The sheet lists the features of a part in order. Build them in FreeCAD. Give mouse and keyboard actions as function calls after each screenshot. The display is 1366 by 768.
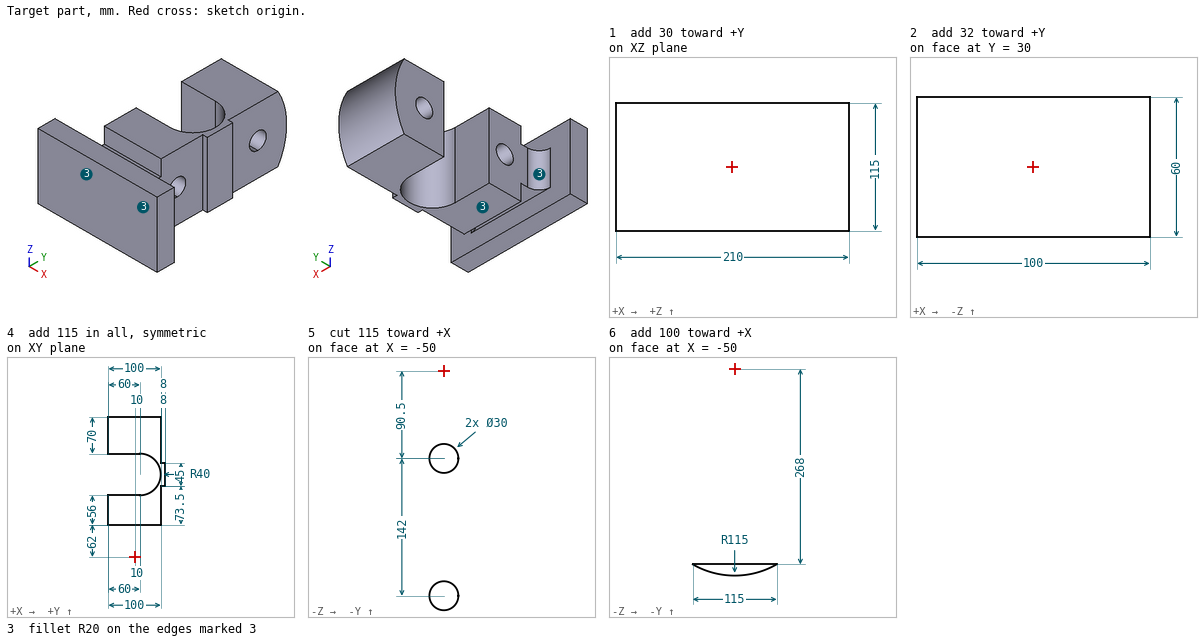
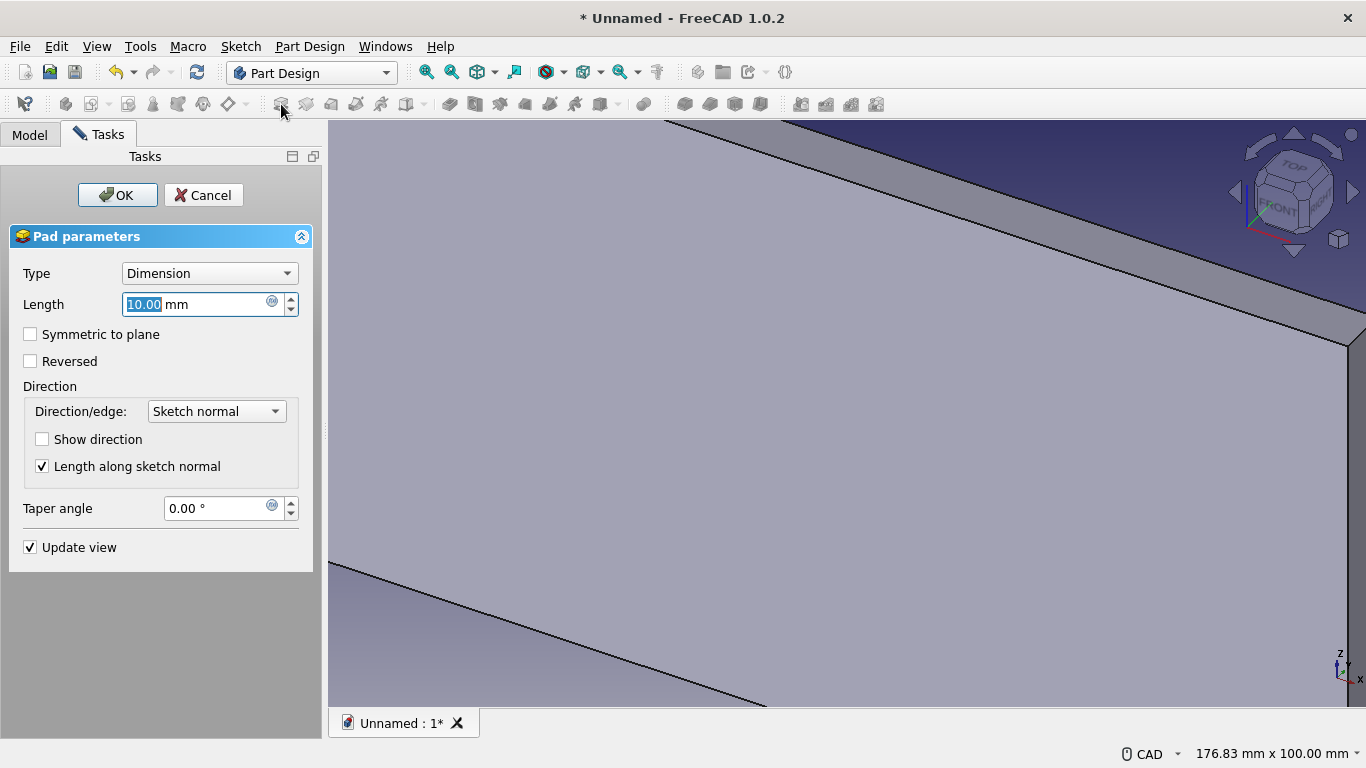
text(30)
key(Tab)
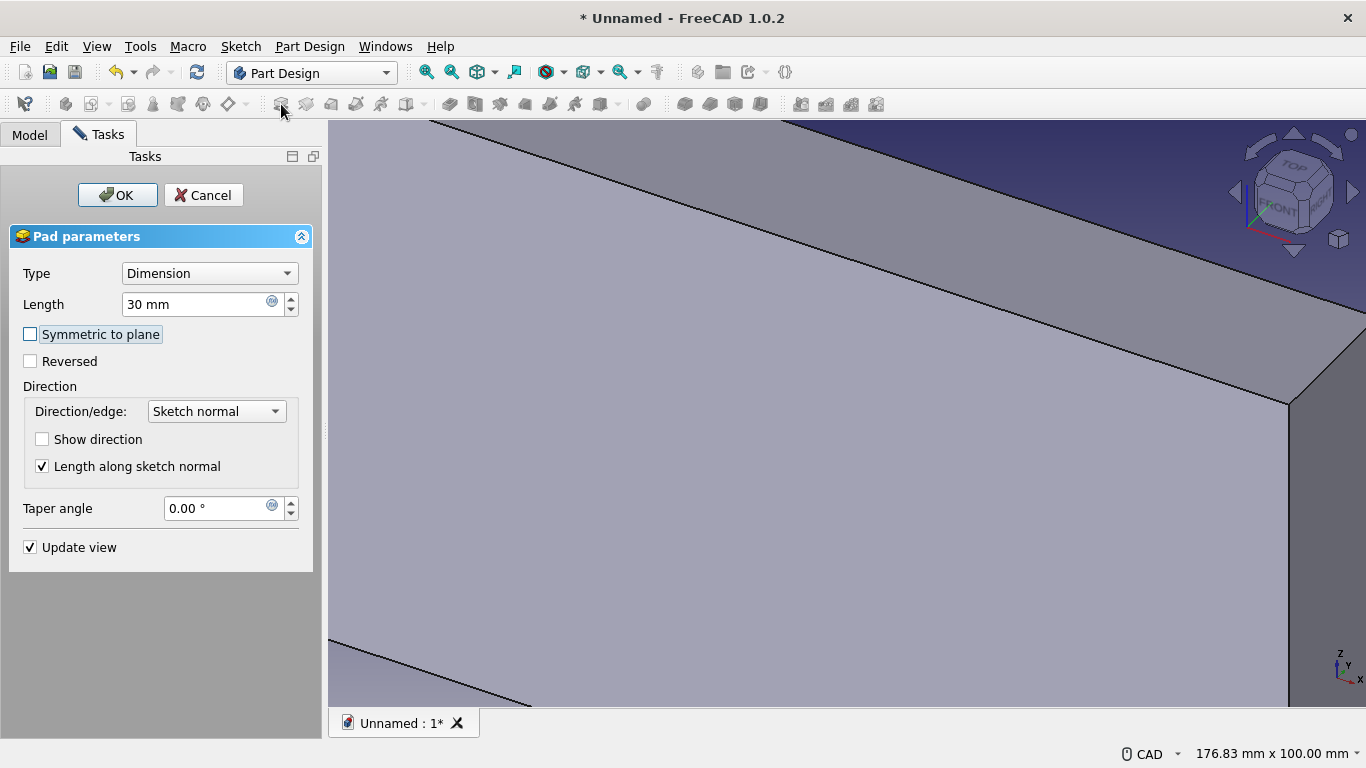
click(31, 361)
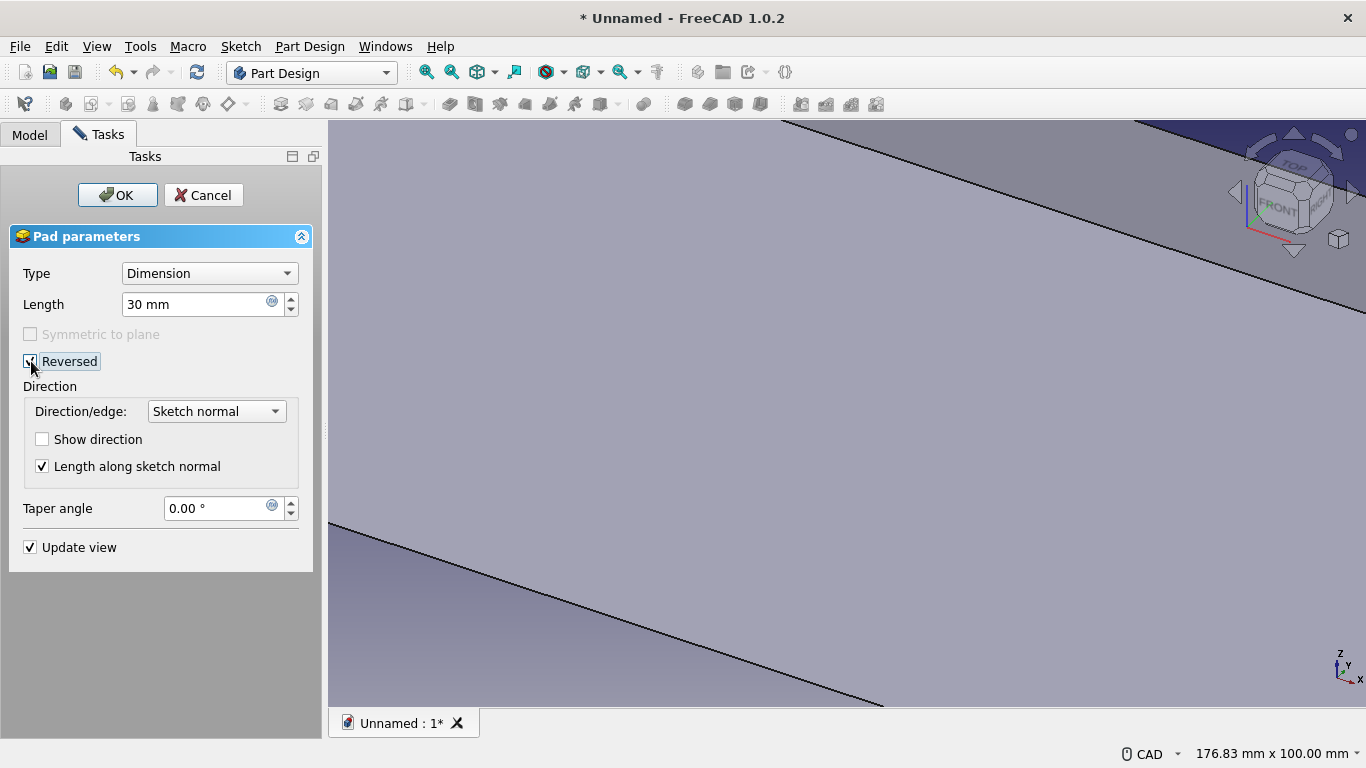
click(118, 195)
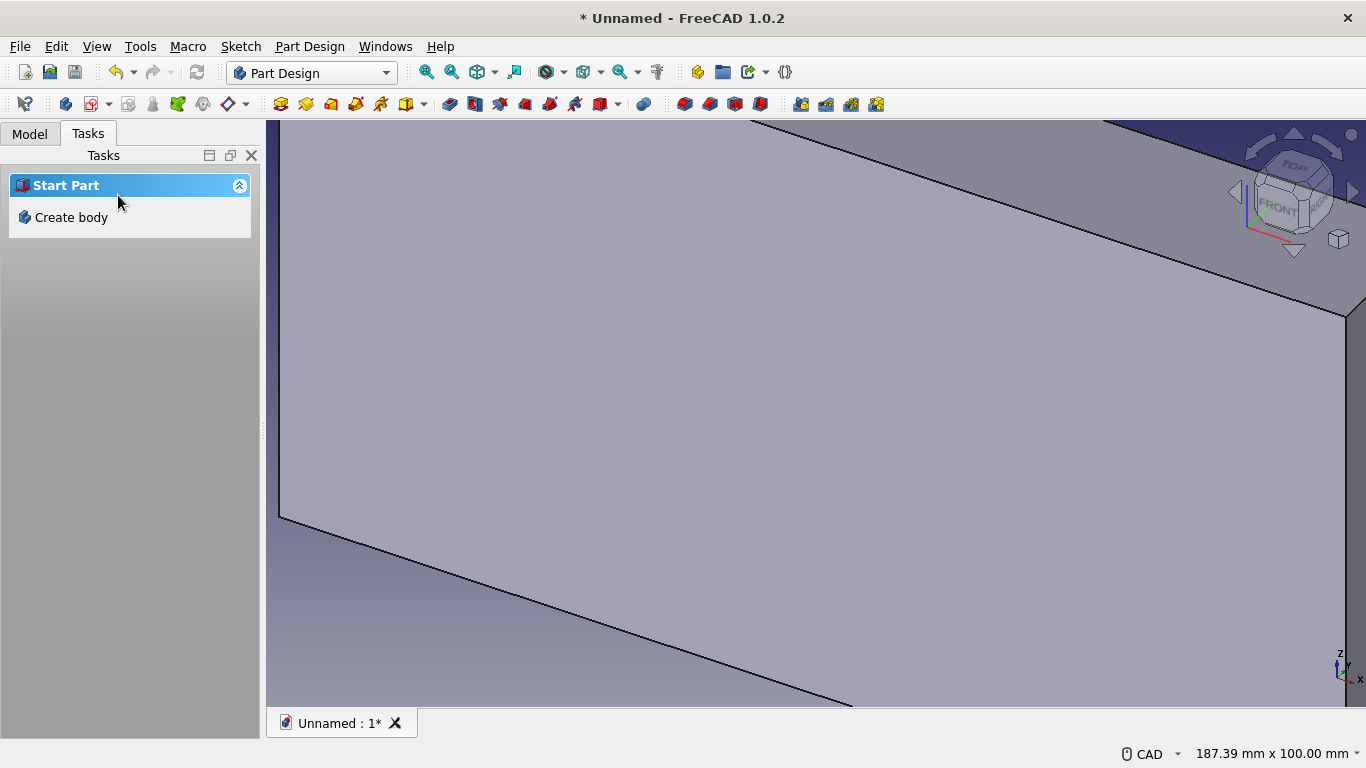
key(v)
key(f)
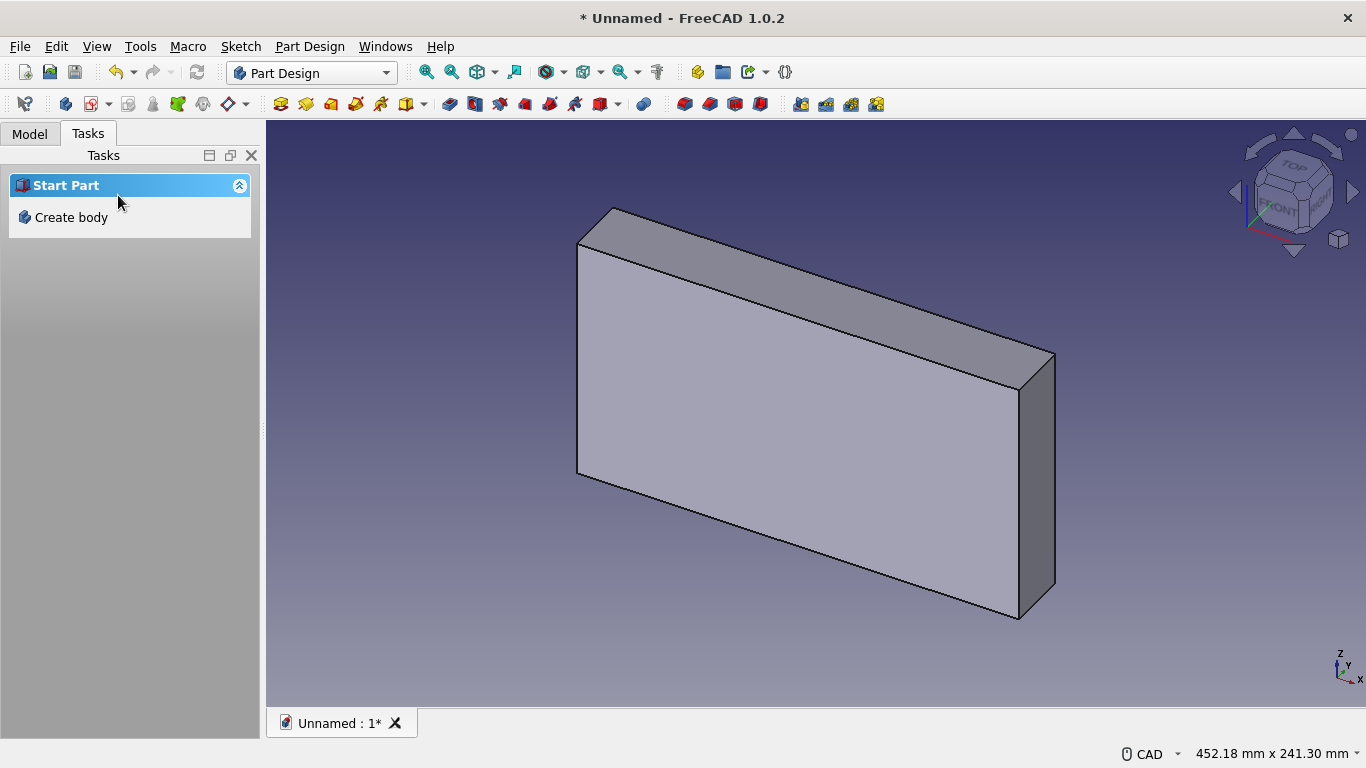
key(4)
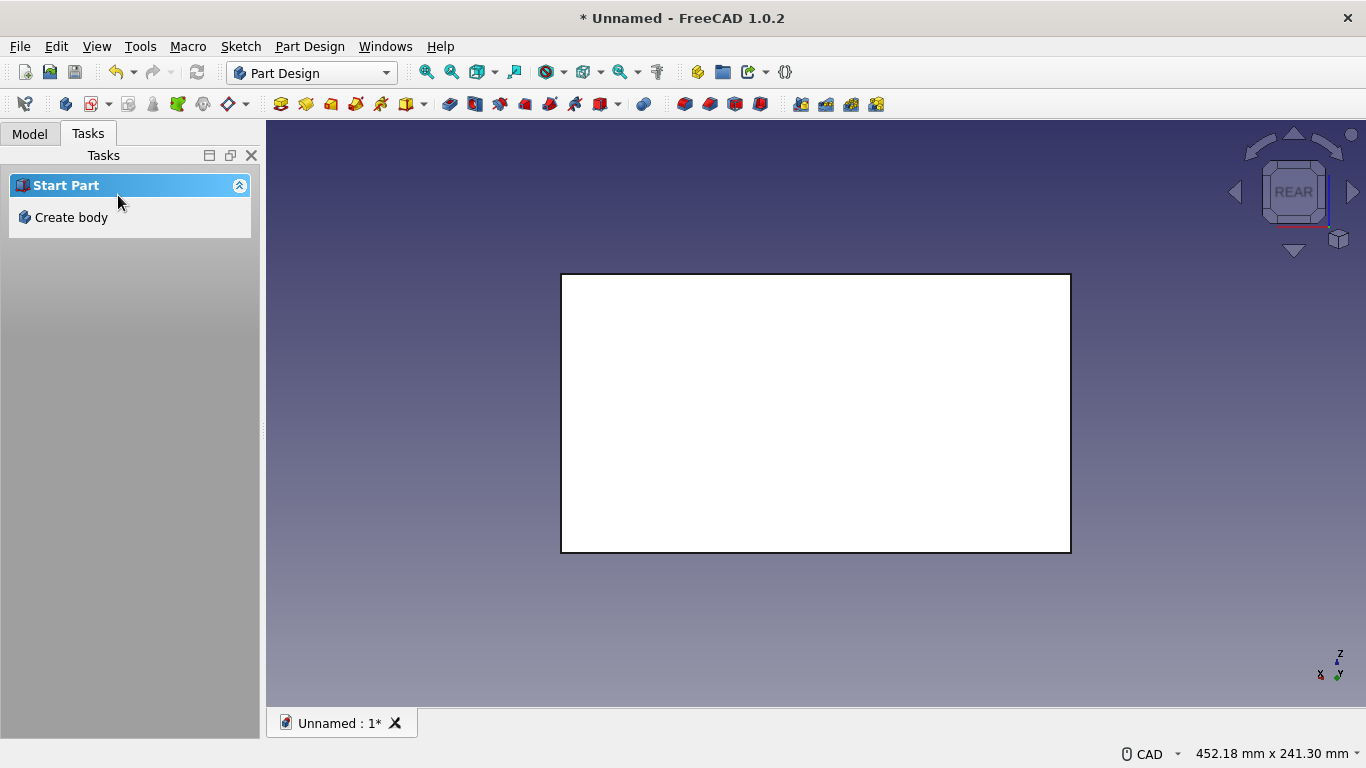
click(743, 413)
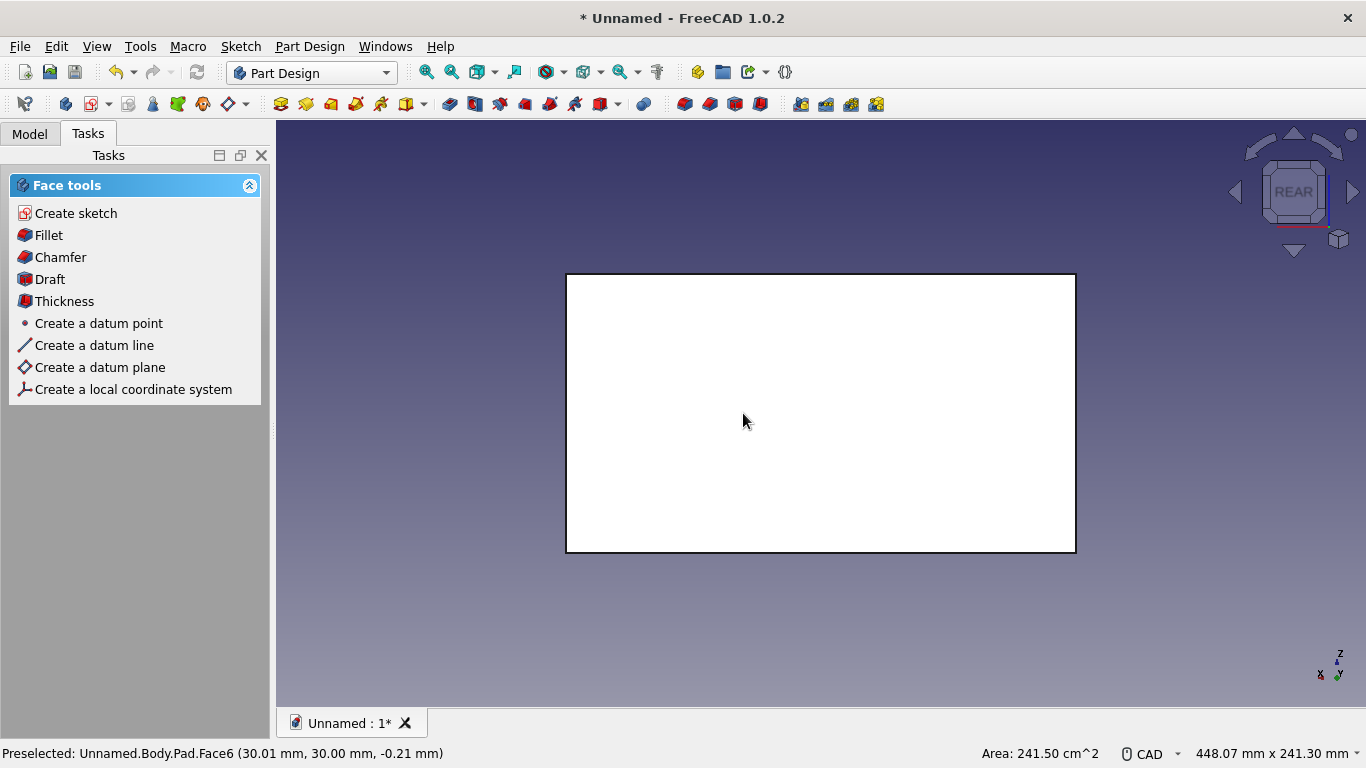
click(90, 104)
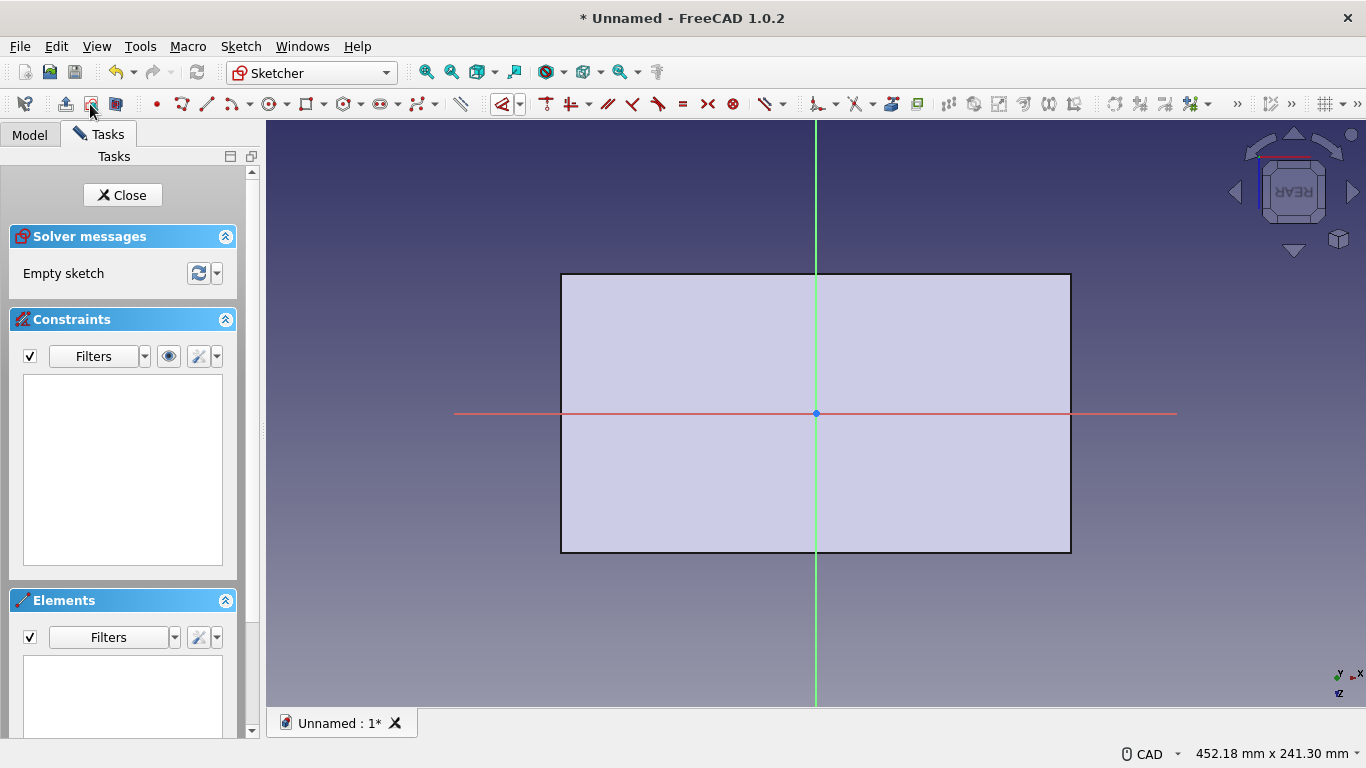
scroll(856, 413, up, 5)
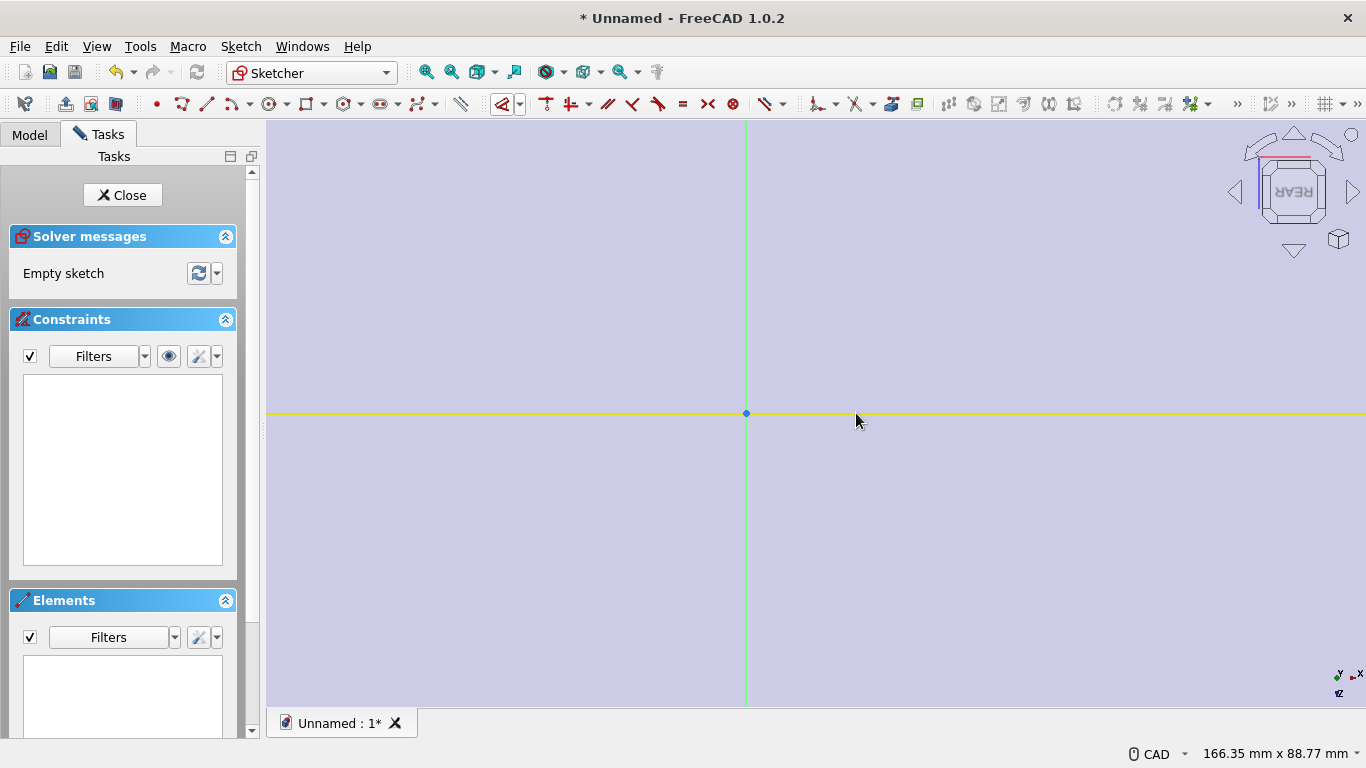
click(324, 104)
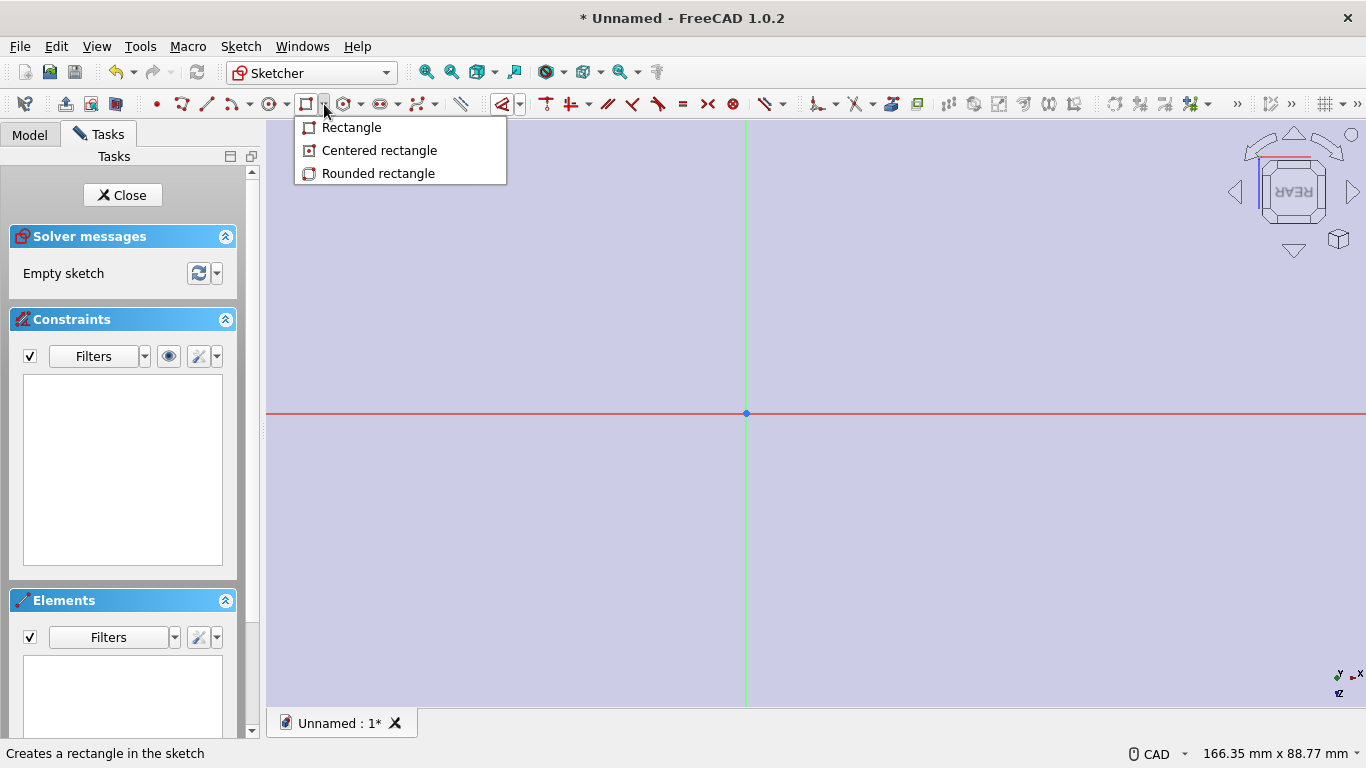
click(400, 150)